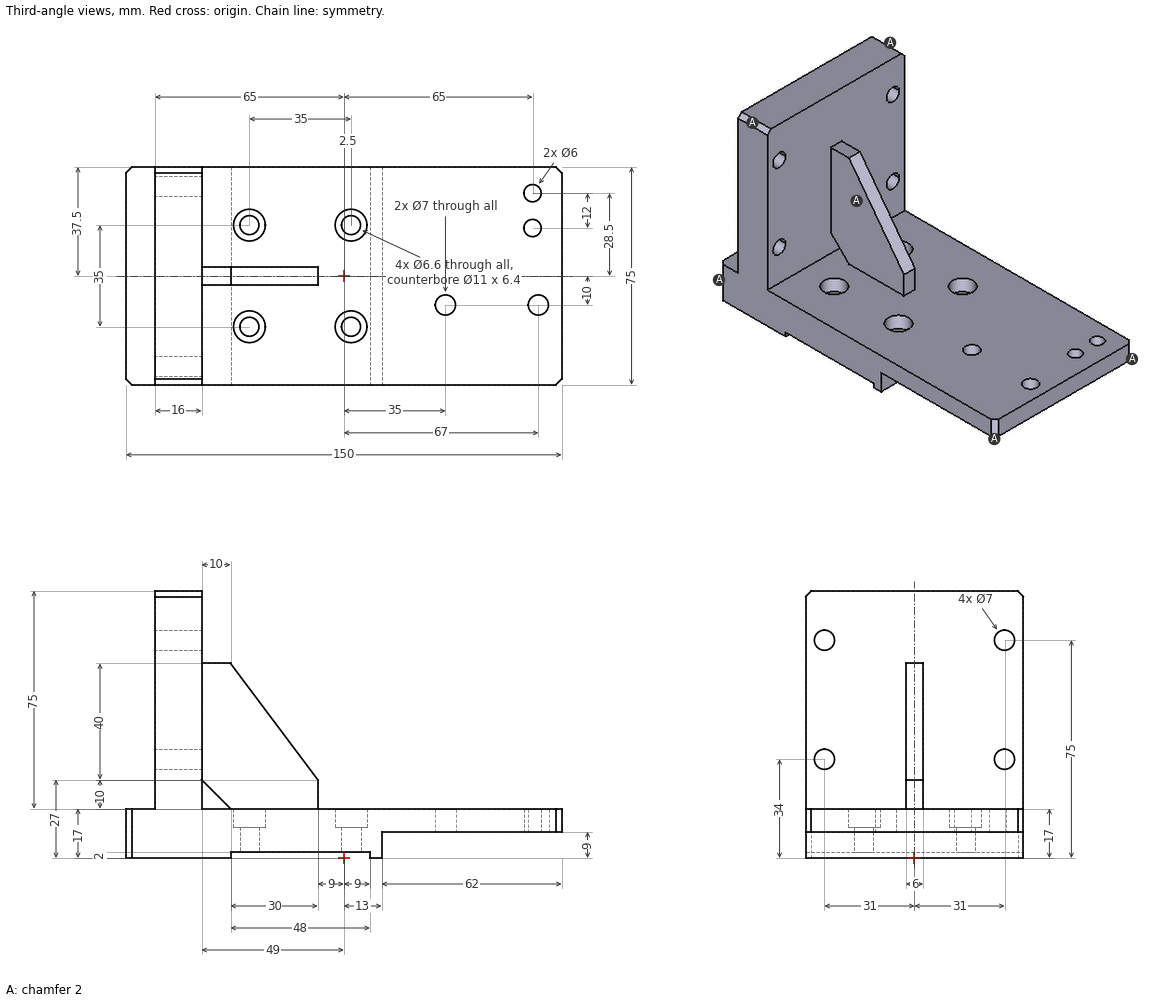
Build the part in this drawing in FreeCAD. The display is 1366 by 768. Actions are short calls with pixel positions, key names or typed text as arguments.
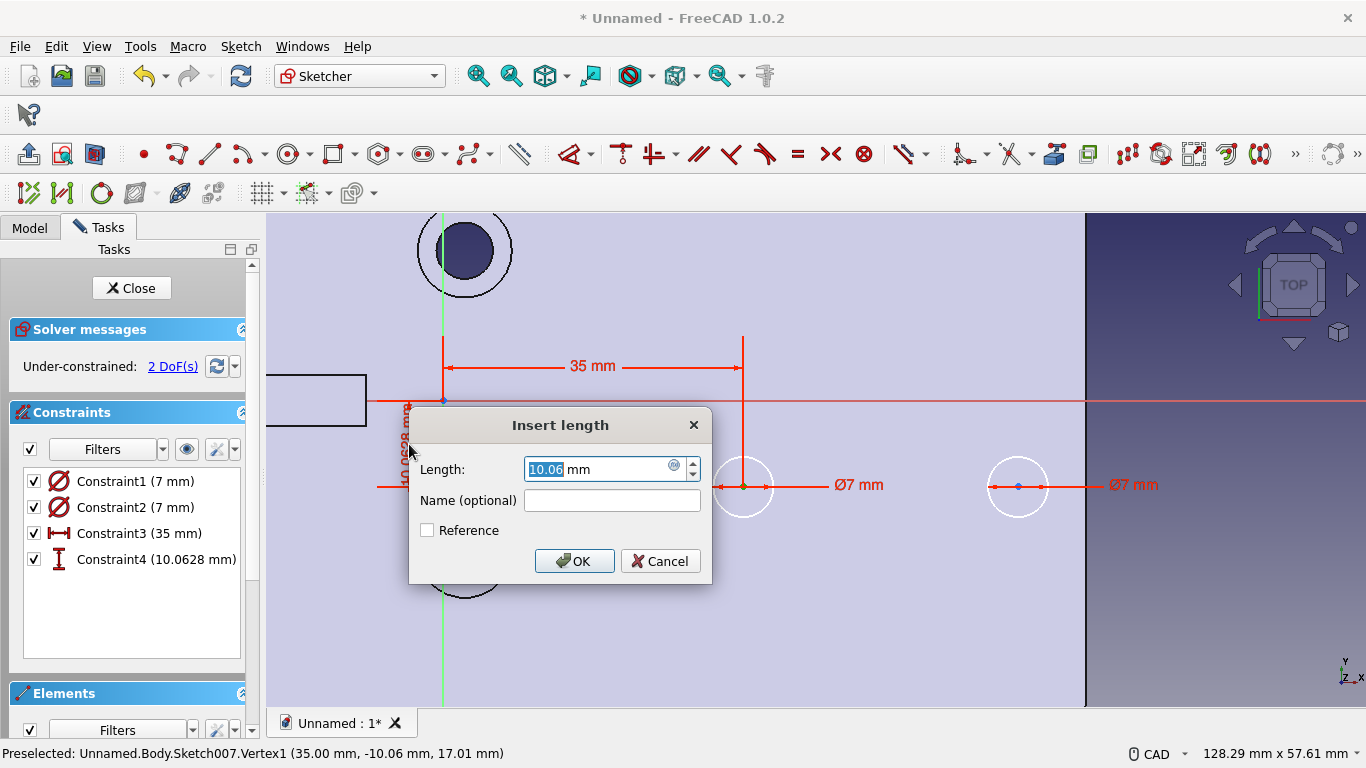
text(10)
key(Return)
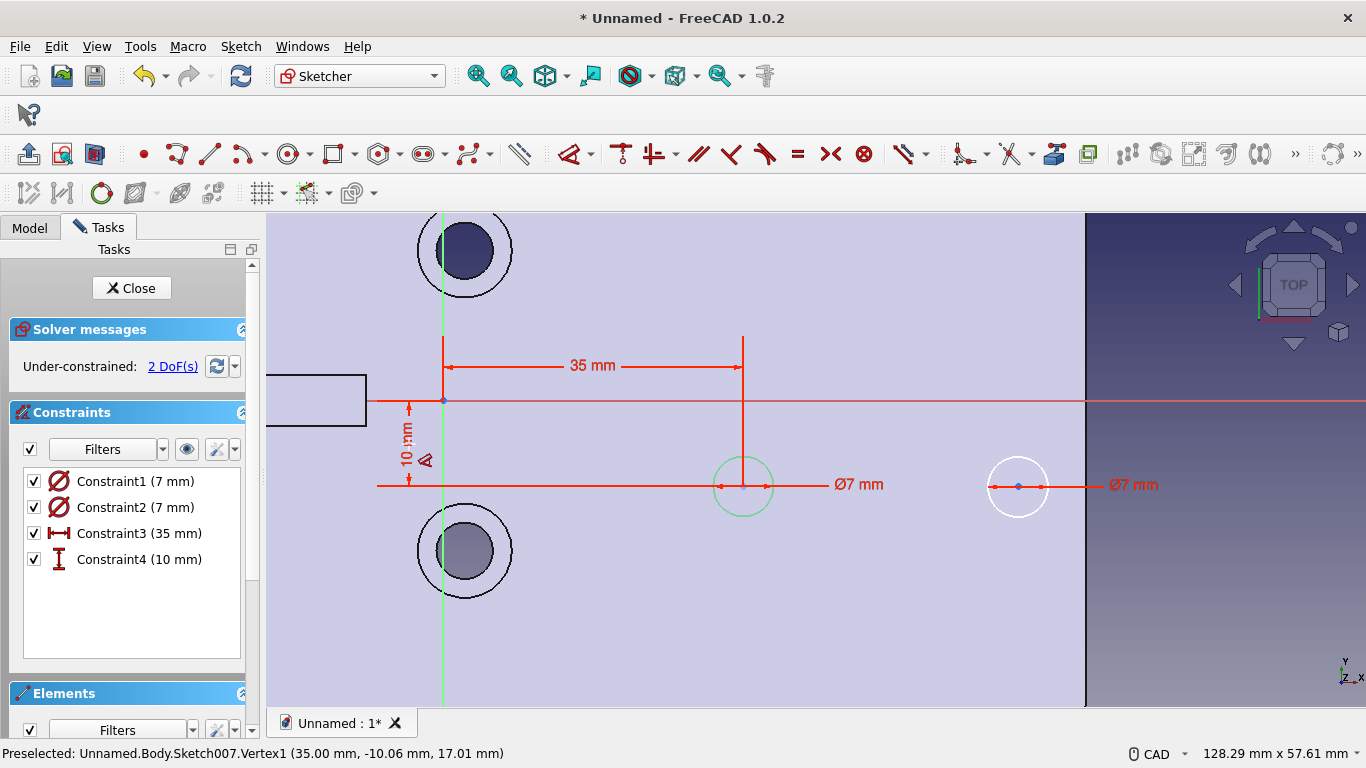
click(1018, 487)
click(731, 367)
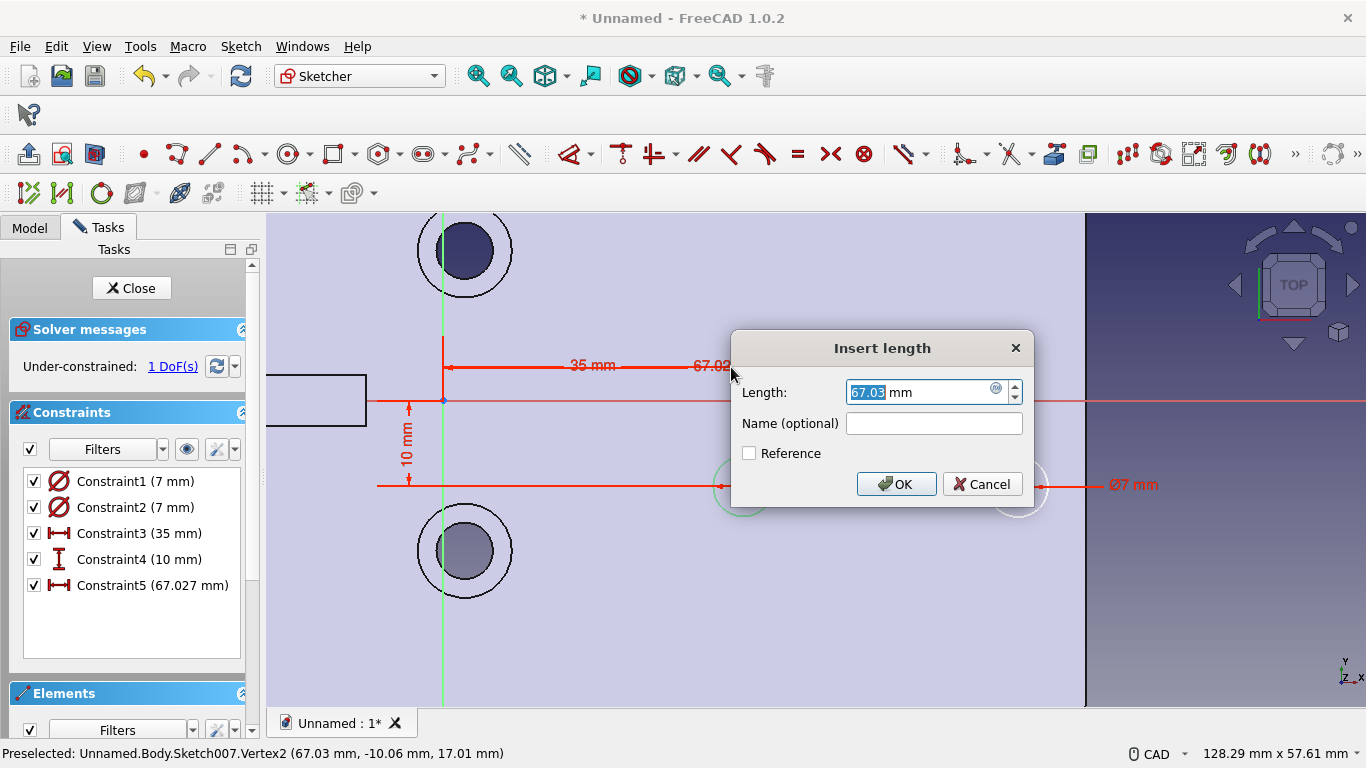
text(67)
key(Return)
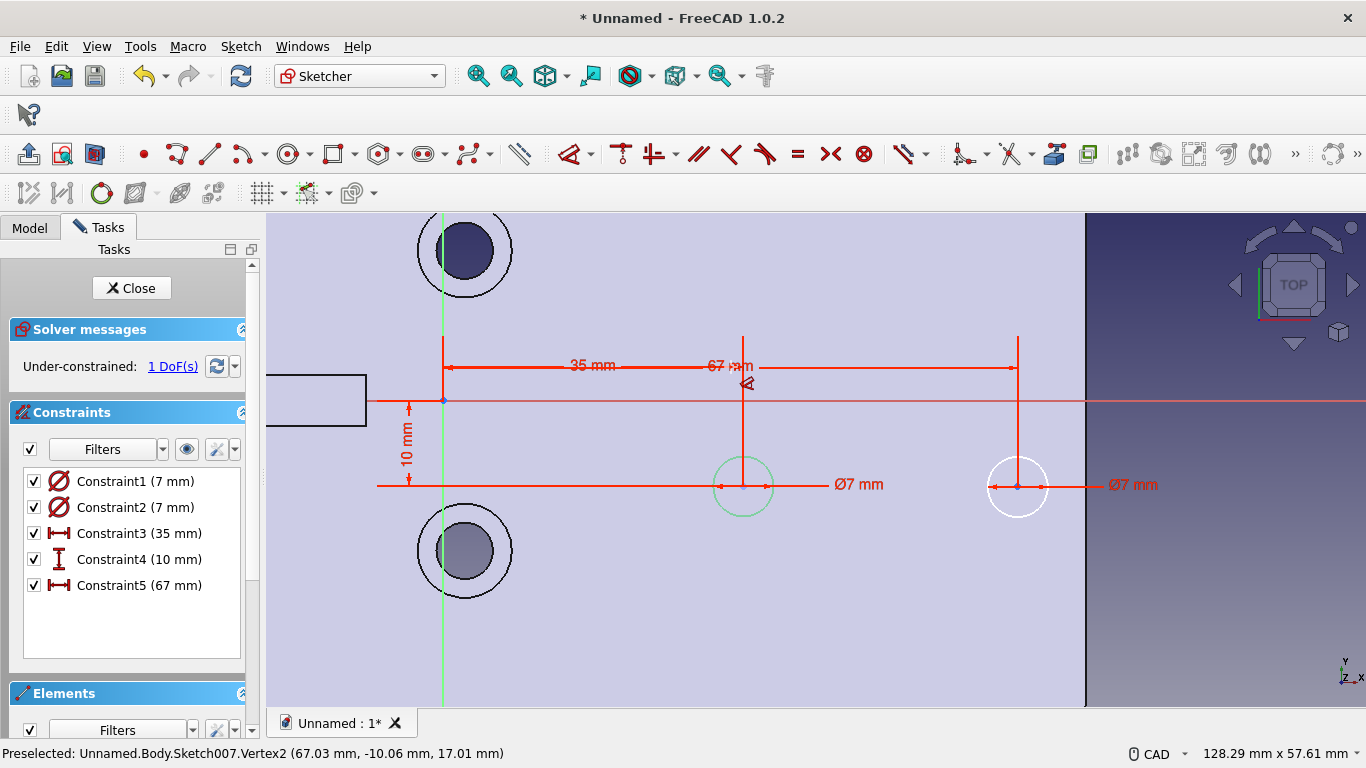
click(1018, 487)
click(409, 474)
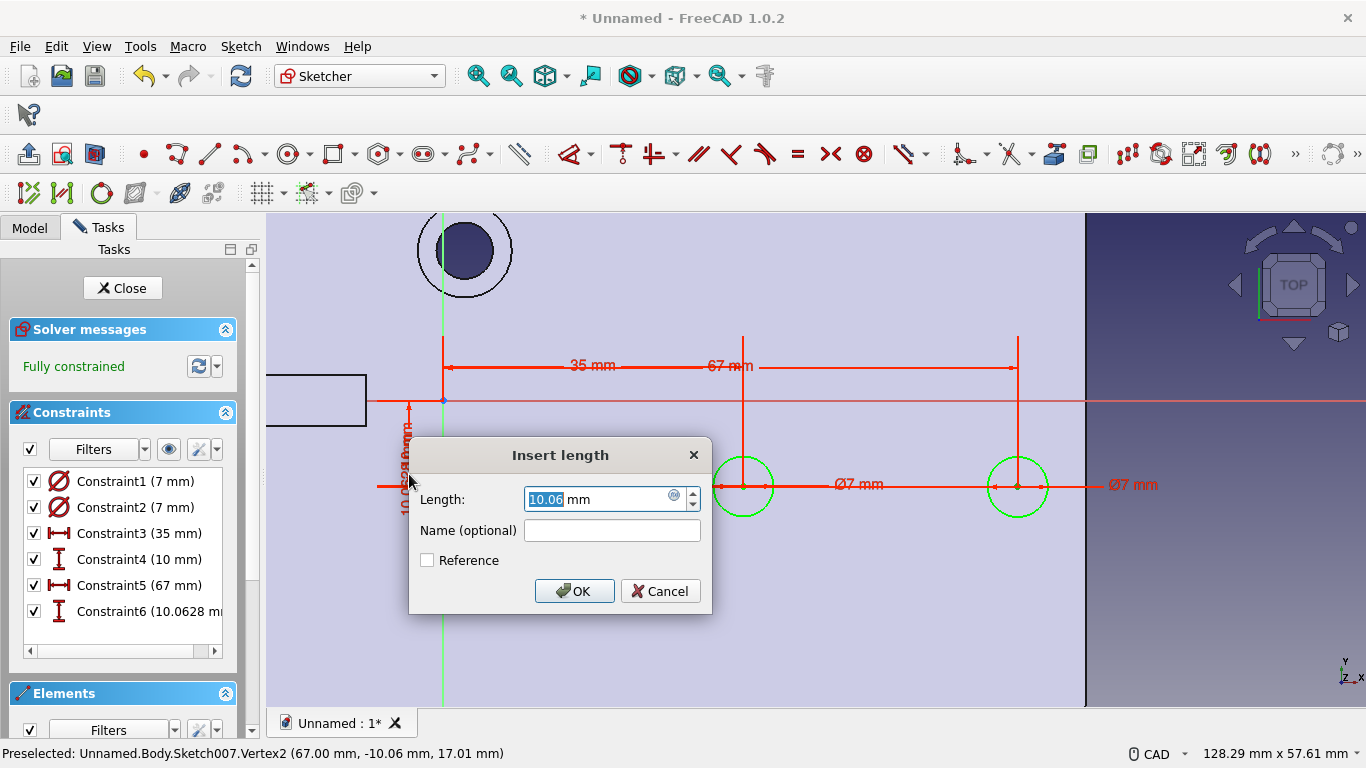
text(10)
key(Return)
key(Escape)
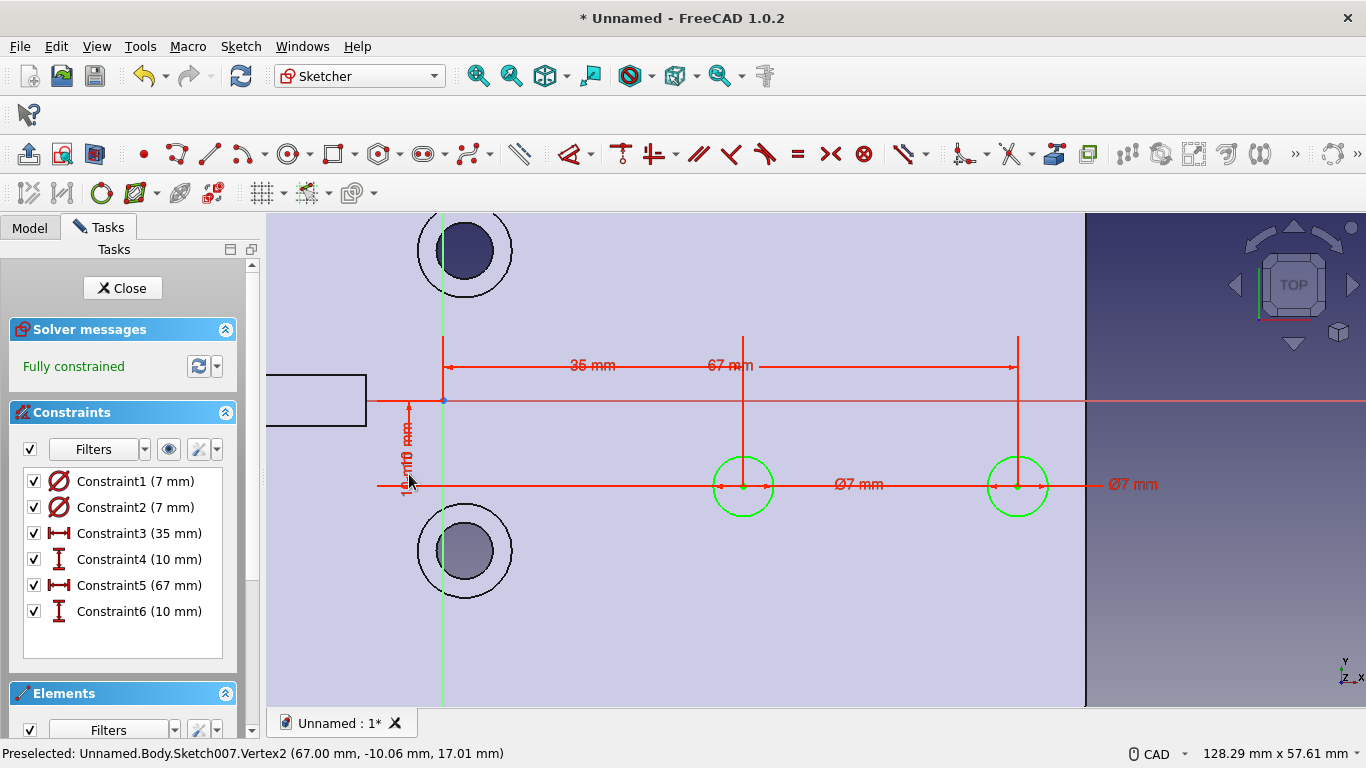
click(123, 288)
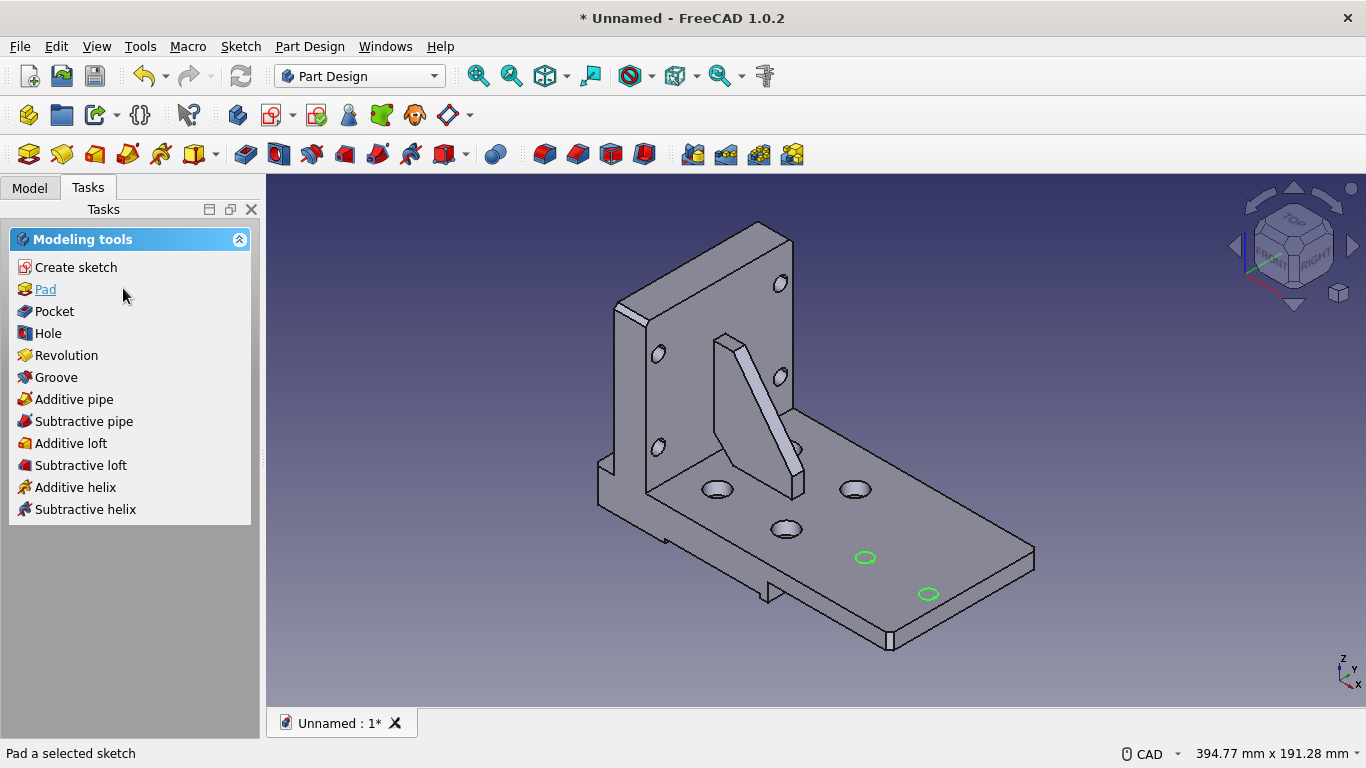
click(279, 154)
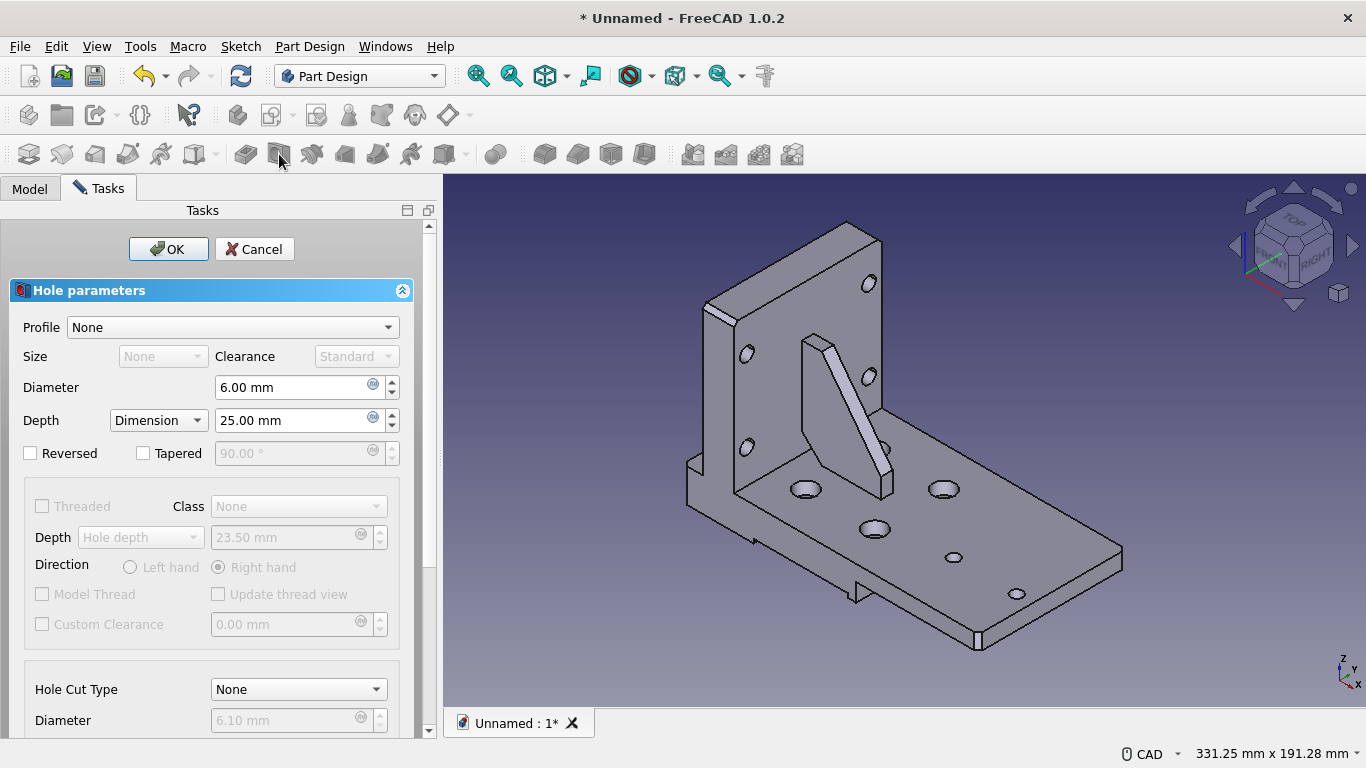
triple_click(300, 388)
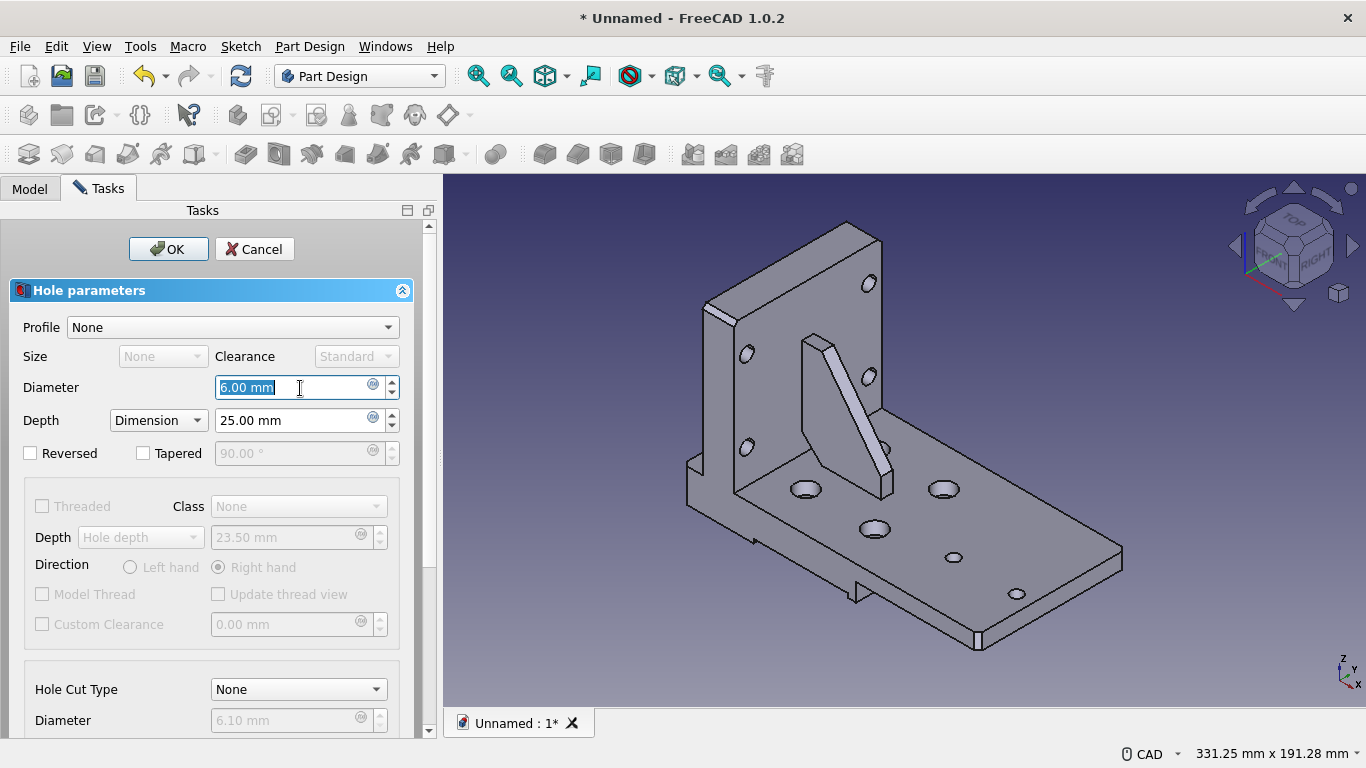
text(7)
key(Tab)